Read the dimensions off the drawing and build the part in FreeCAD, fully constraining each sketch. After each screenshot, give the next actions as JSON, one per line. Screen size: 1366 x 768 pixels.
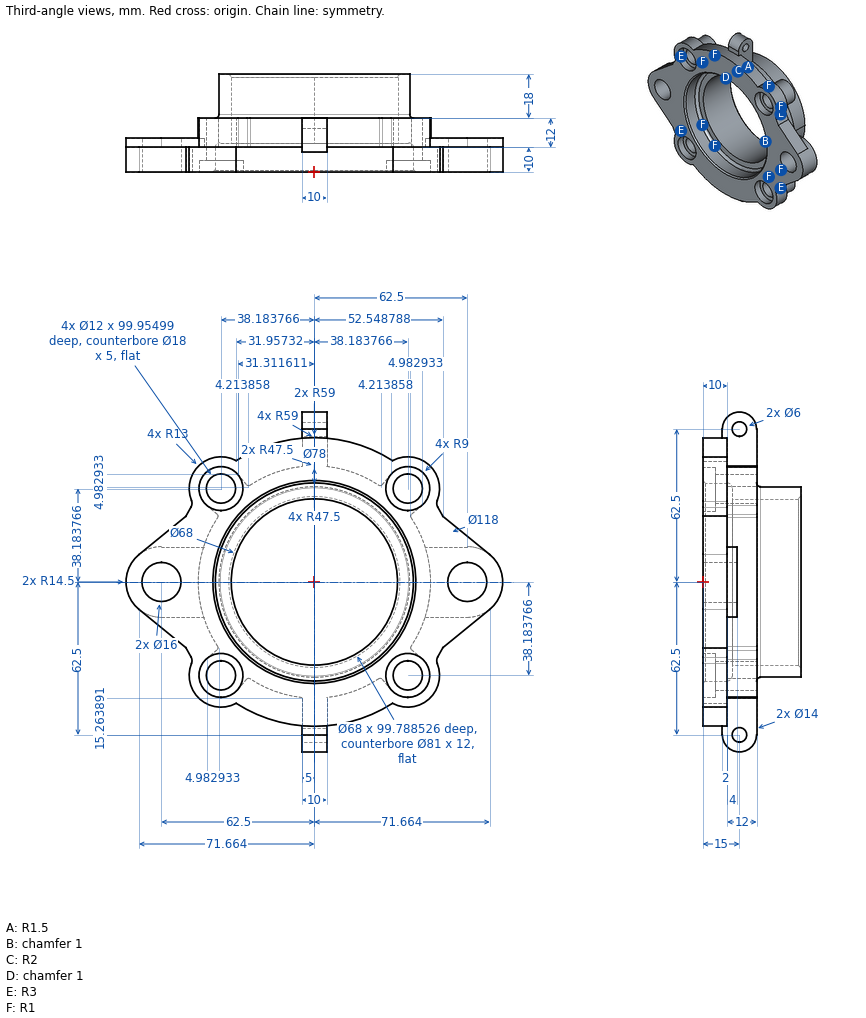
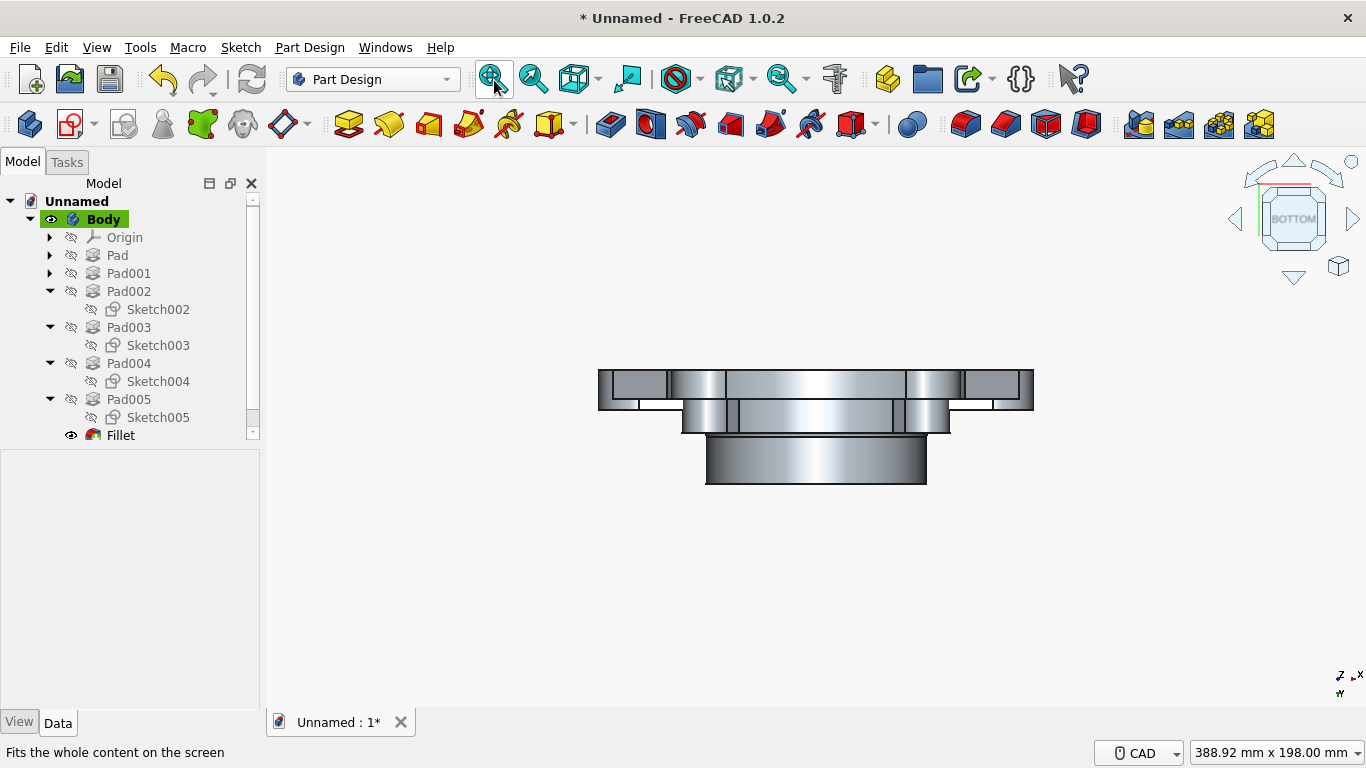
{"action": "left_click", "coordinate": [494, 80]}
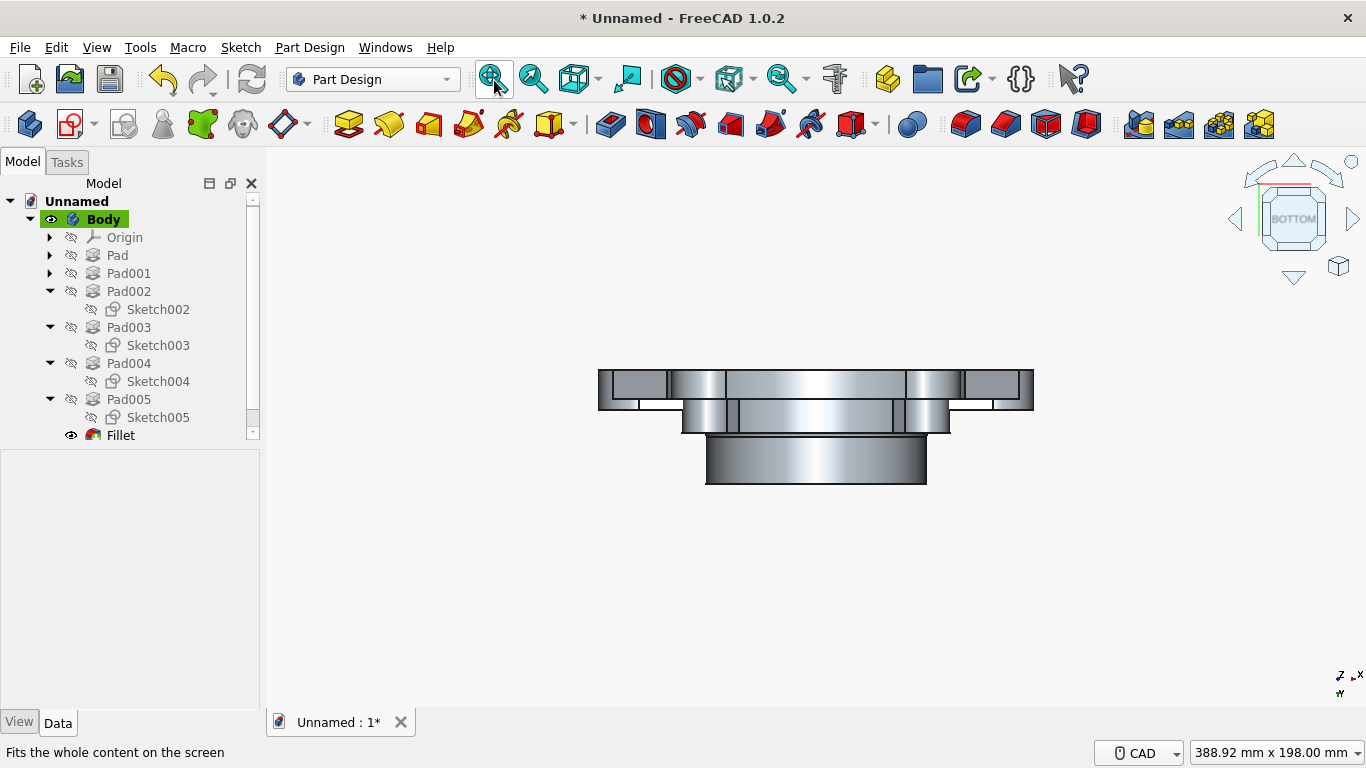
{"action": "key", "text": "4"}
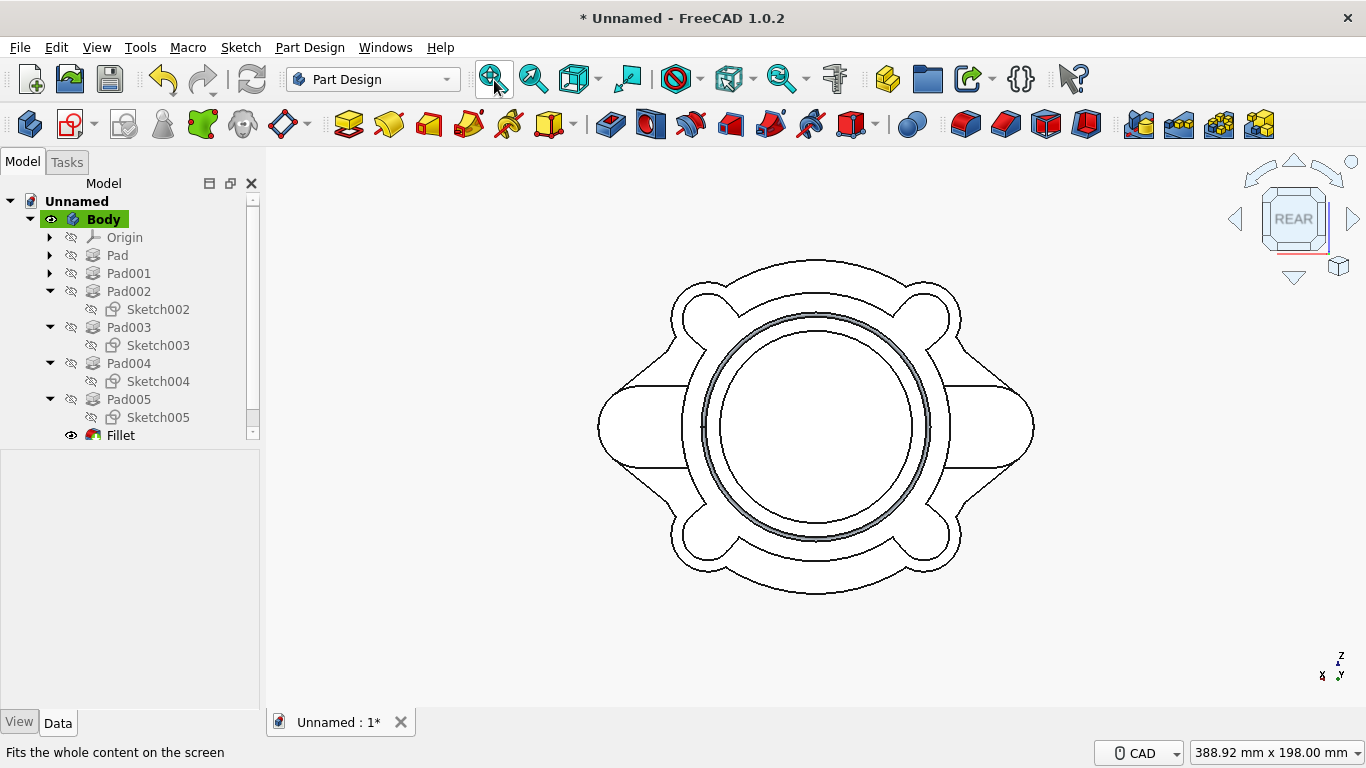
{"action": "left_click", "coordinate": [912, 426]}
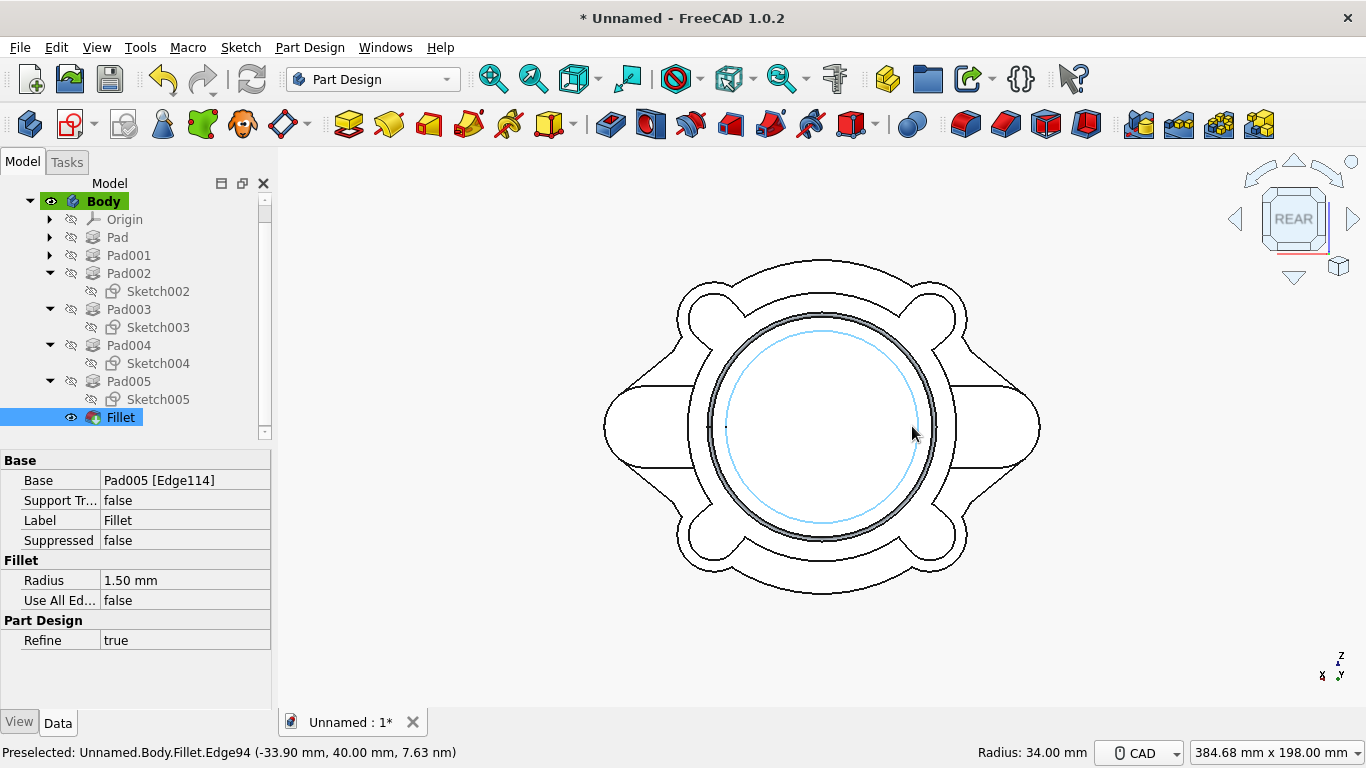
{"action": "left_click", "coordinate": [1006, 124]}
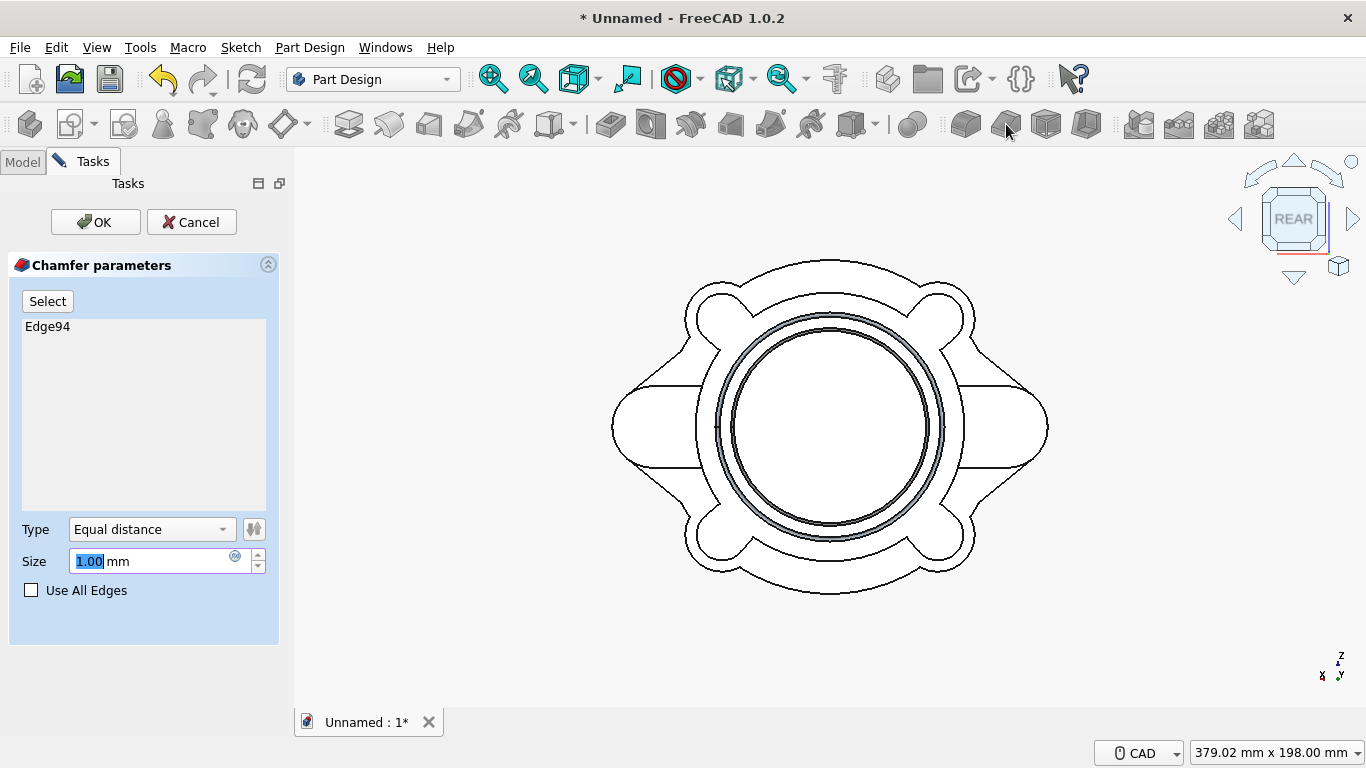
{"action": "type", "text": "1"}
{"action": "key", "text": "Tab"}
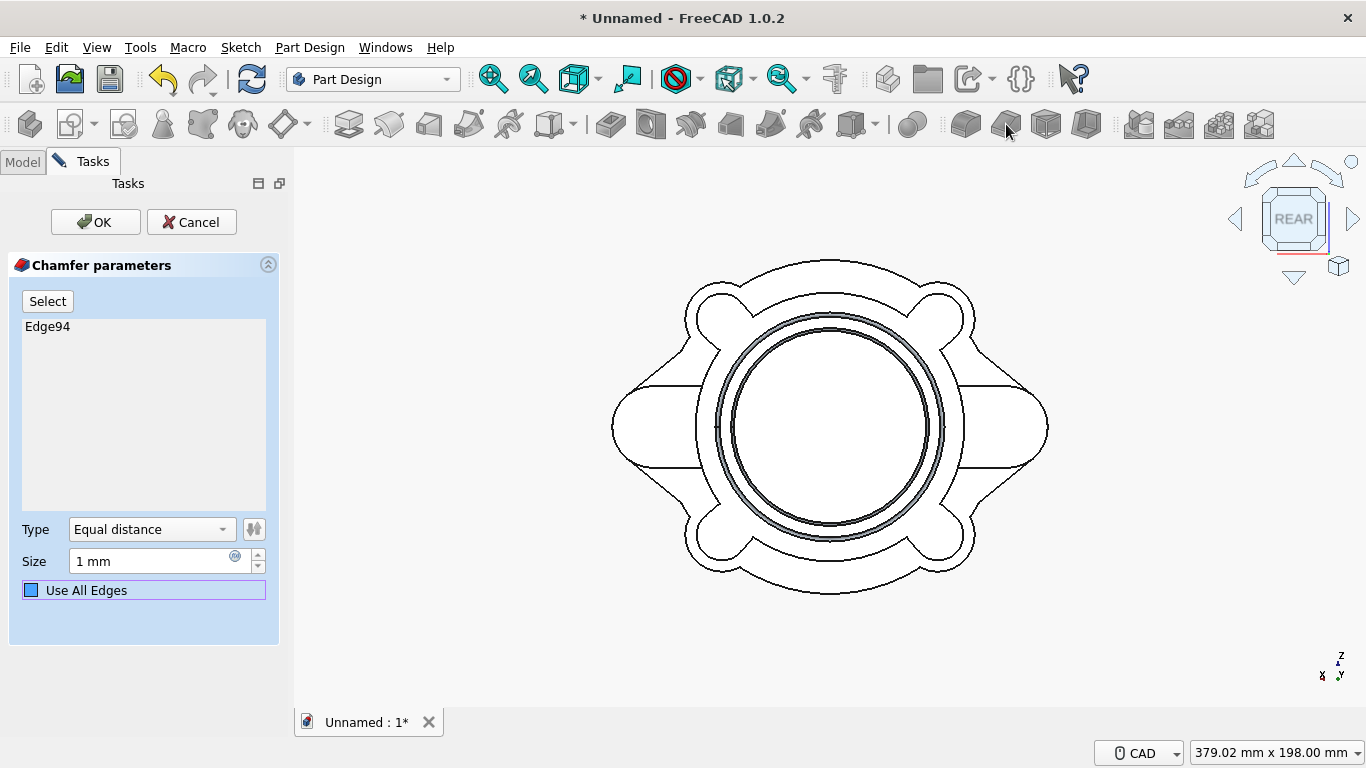
{"action": "left_click", "coordinate": [96, 222]}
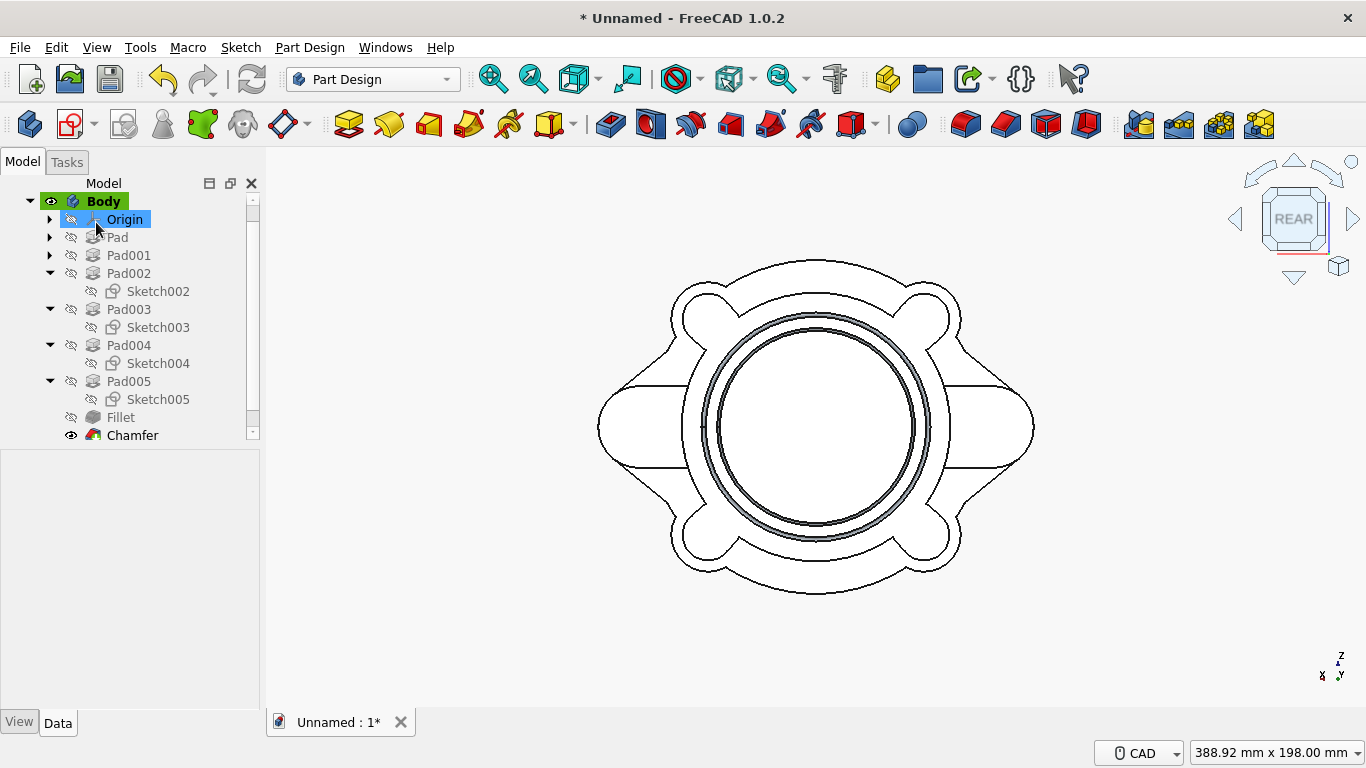
{"action": "left_click", "coordinate": [643, 426]}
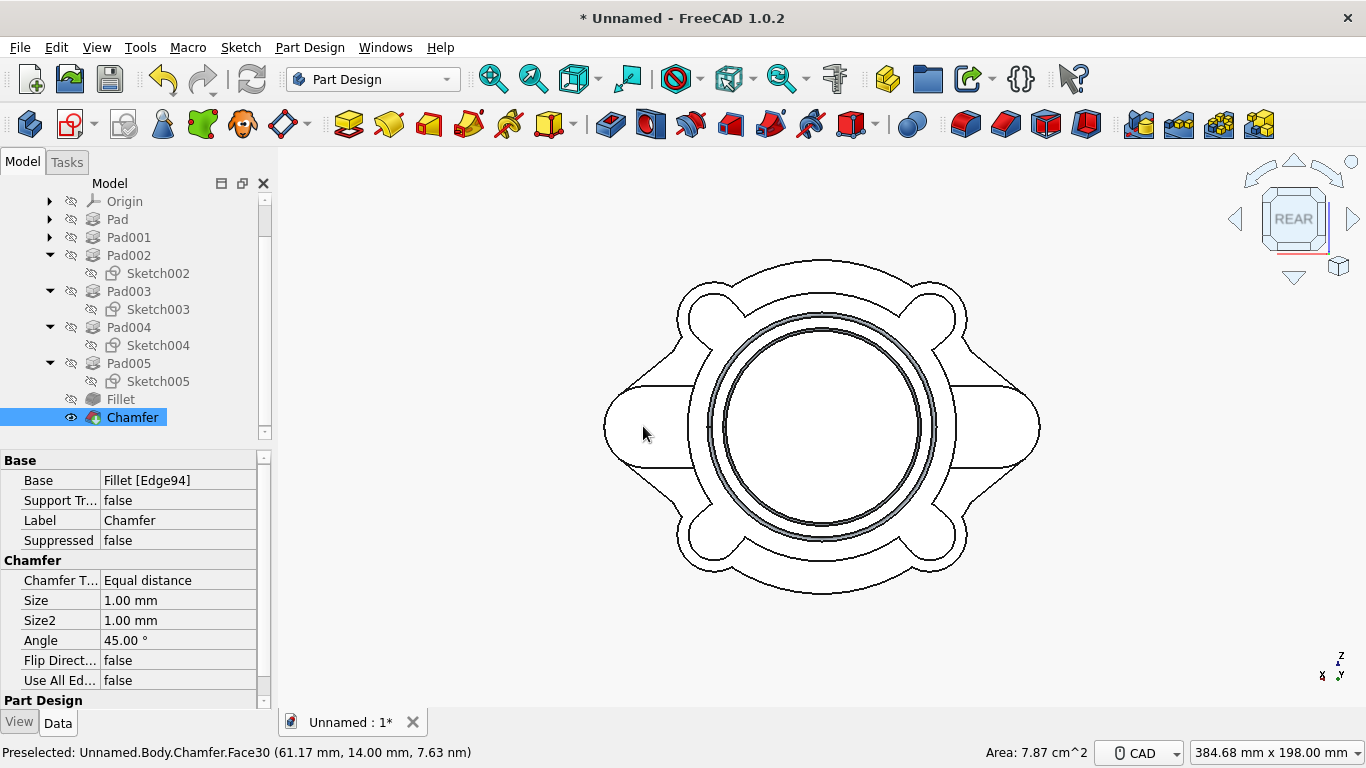
{"action": "left_click", "coordinate": [70, 124]}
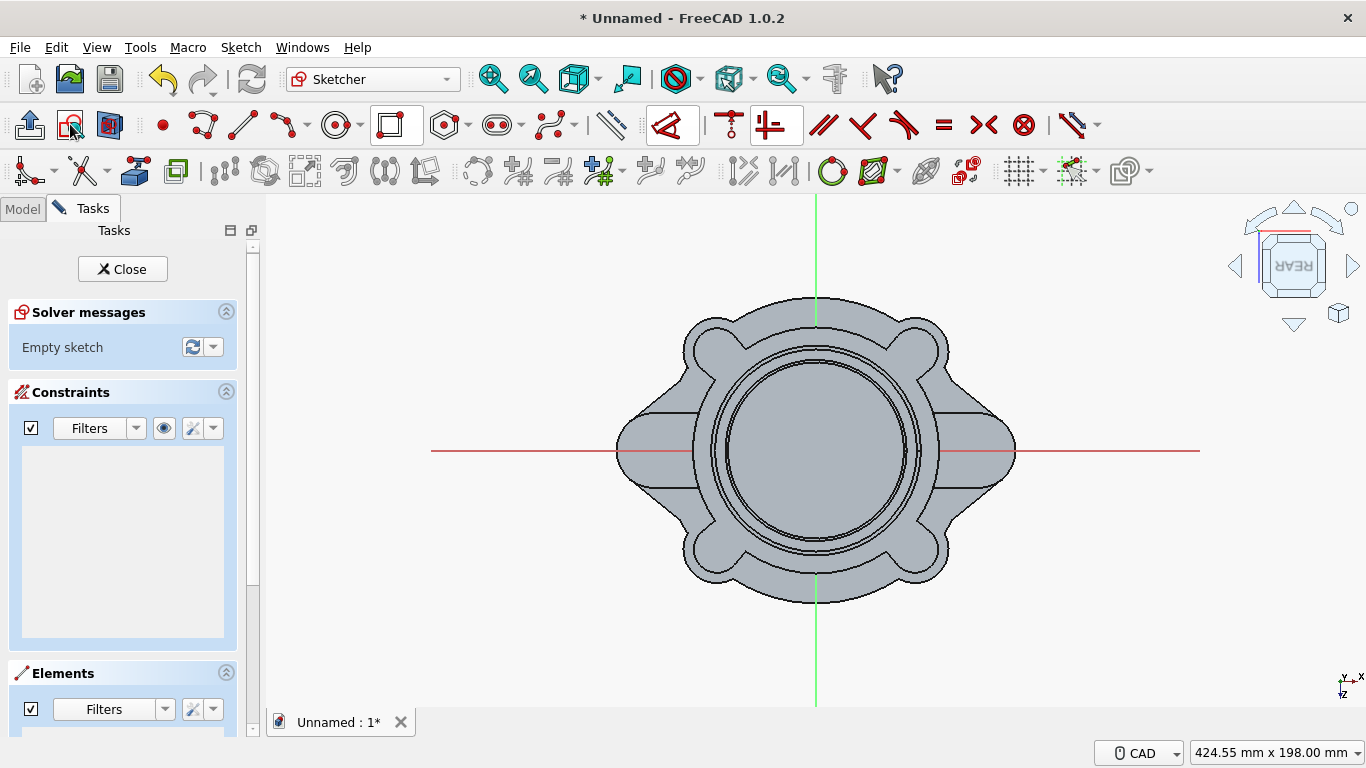
{"action": "scroll", "coordinate": [899, 450], "scroll_direction": "up", "scroll_amount": 3}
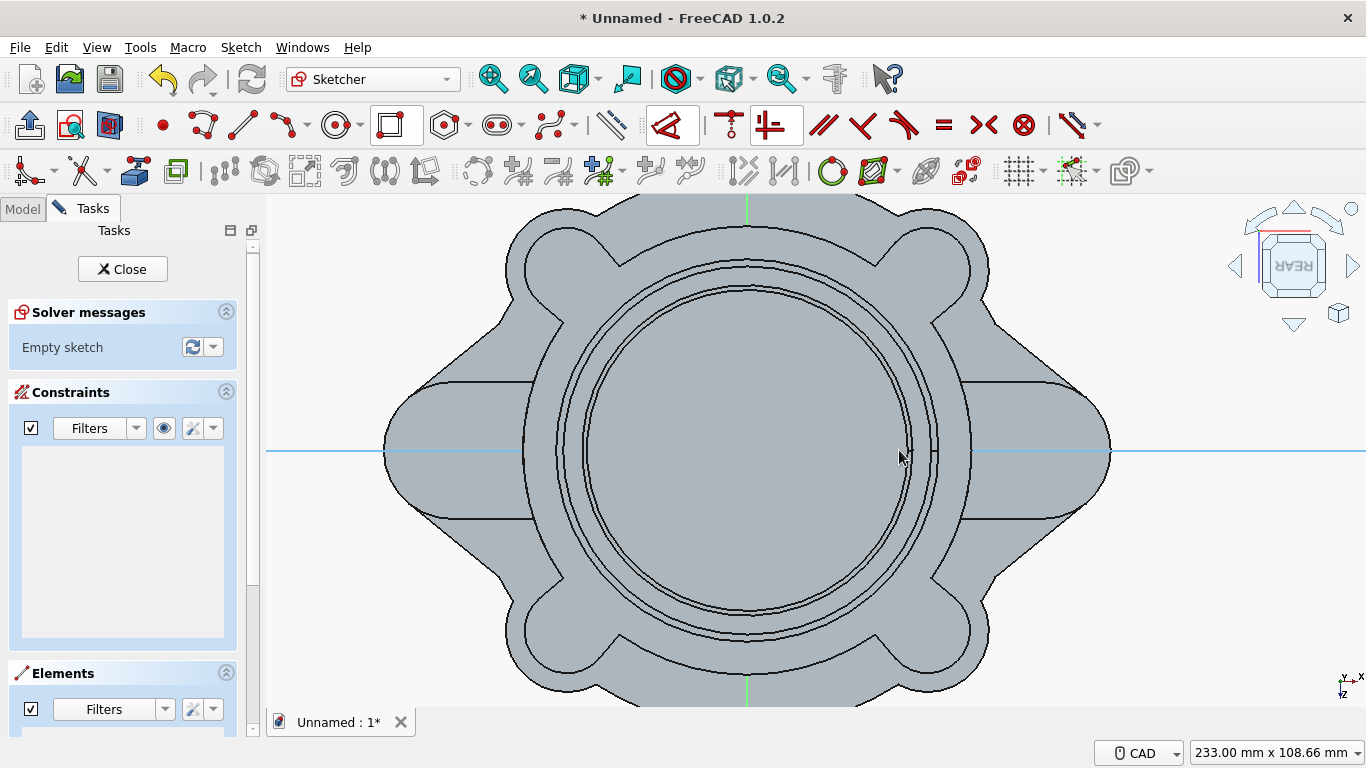
{"action": "left_click", "coordinate": [336, 126]}